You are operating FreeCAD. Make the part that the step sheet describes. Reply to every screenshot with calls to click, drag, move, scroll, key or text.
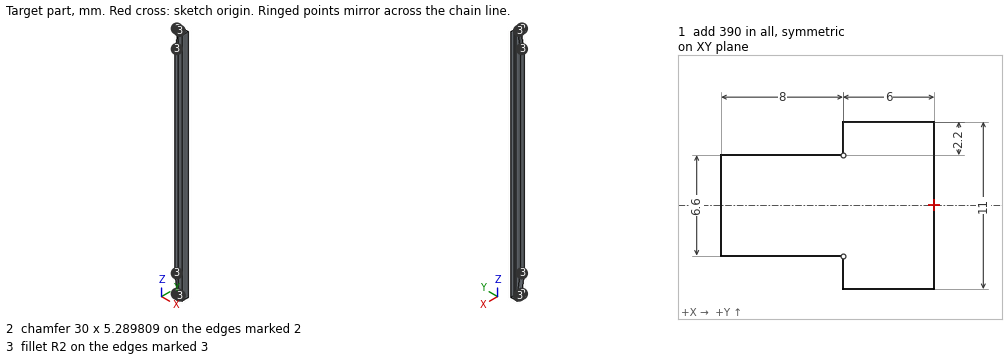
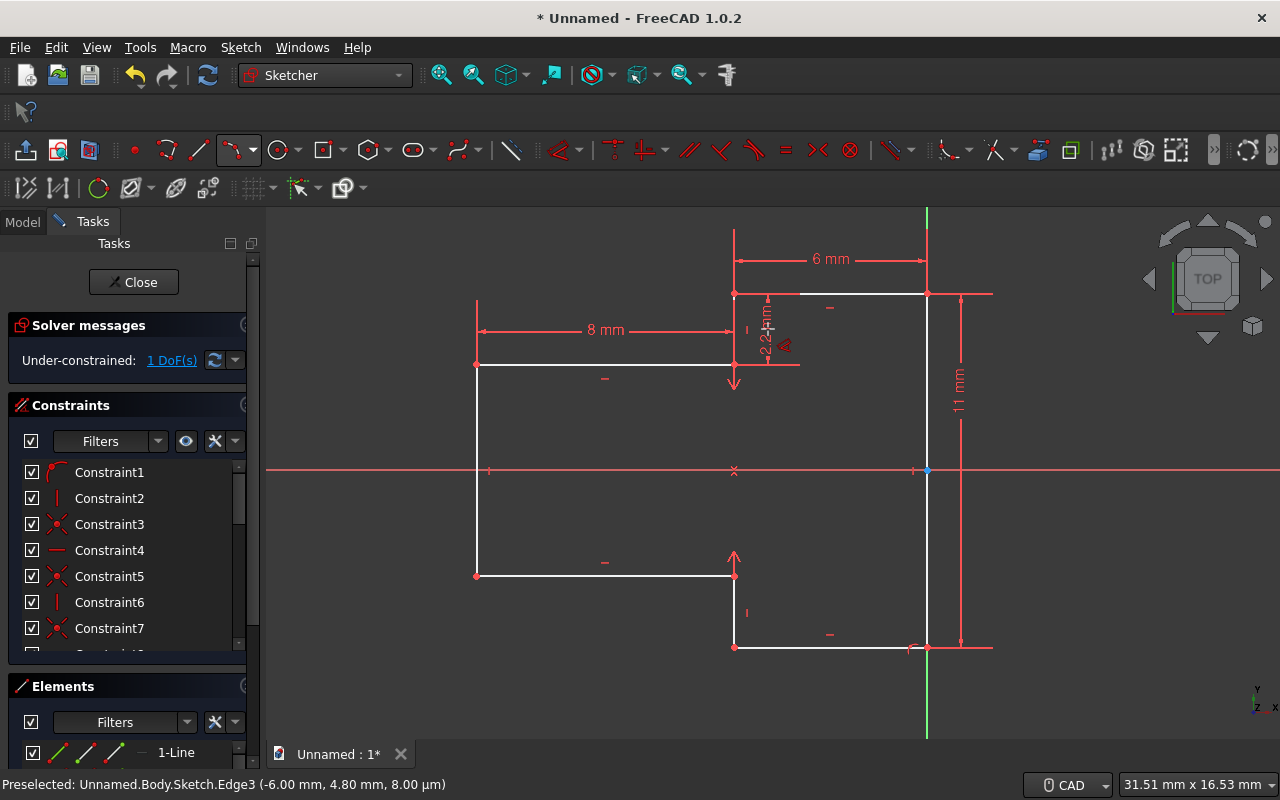
click(477, 428)
click(443, 422)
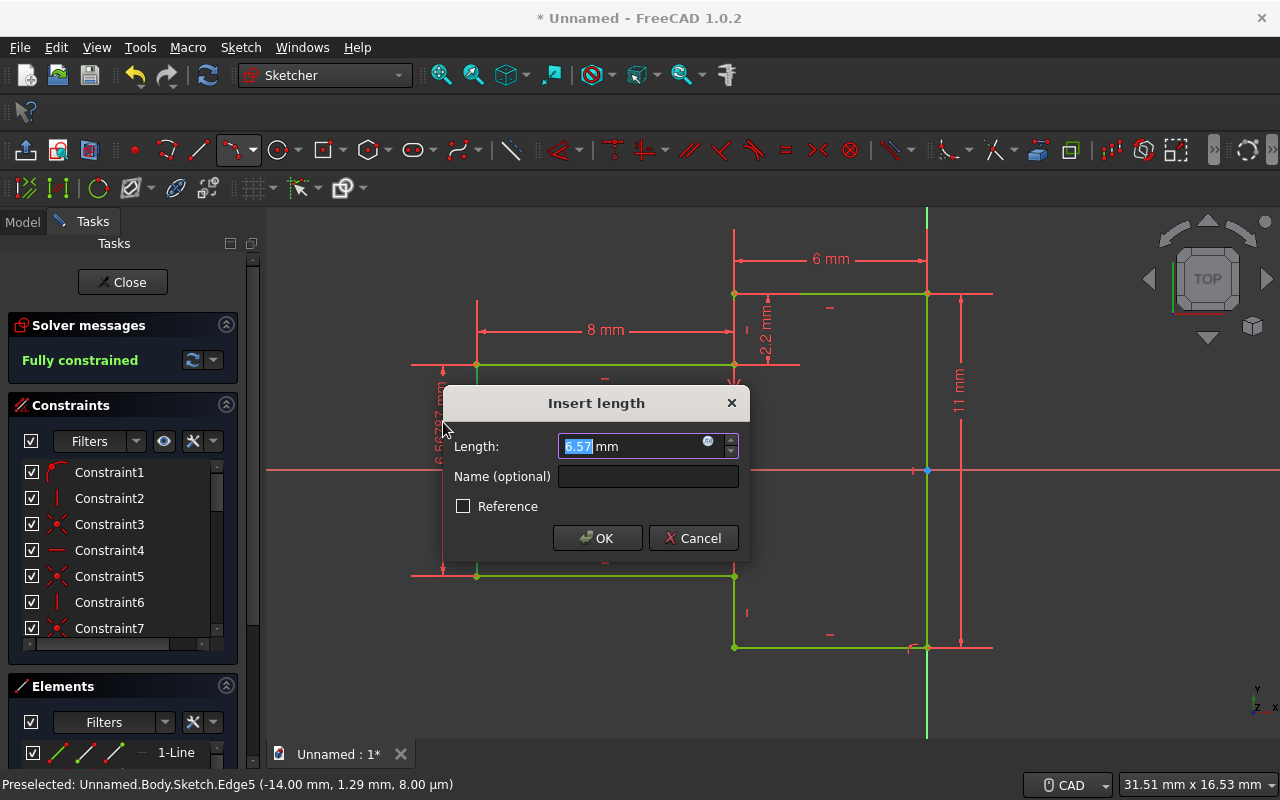
text(6.6)
key(Return)
key(Escape)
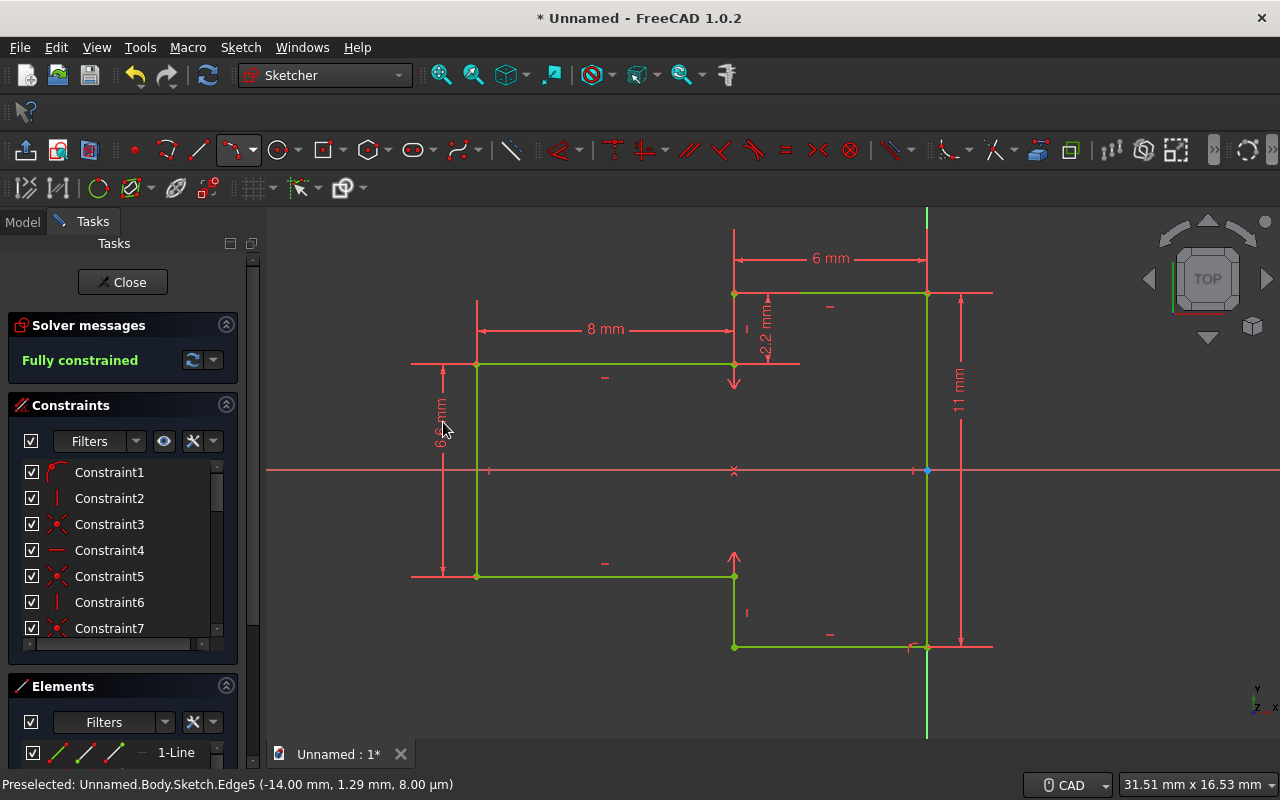
click(123, 282)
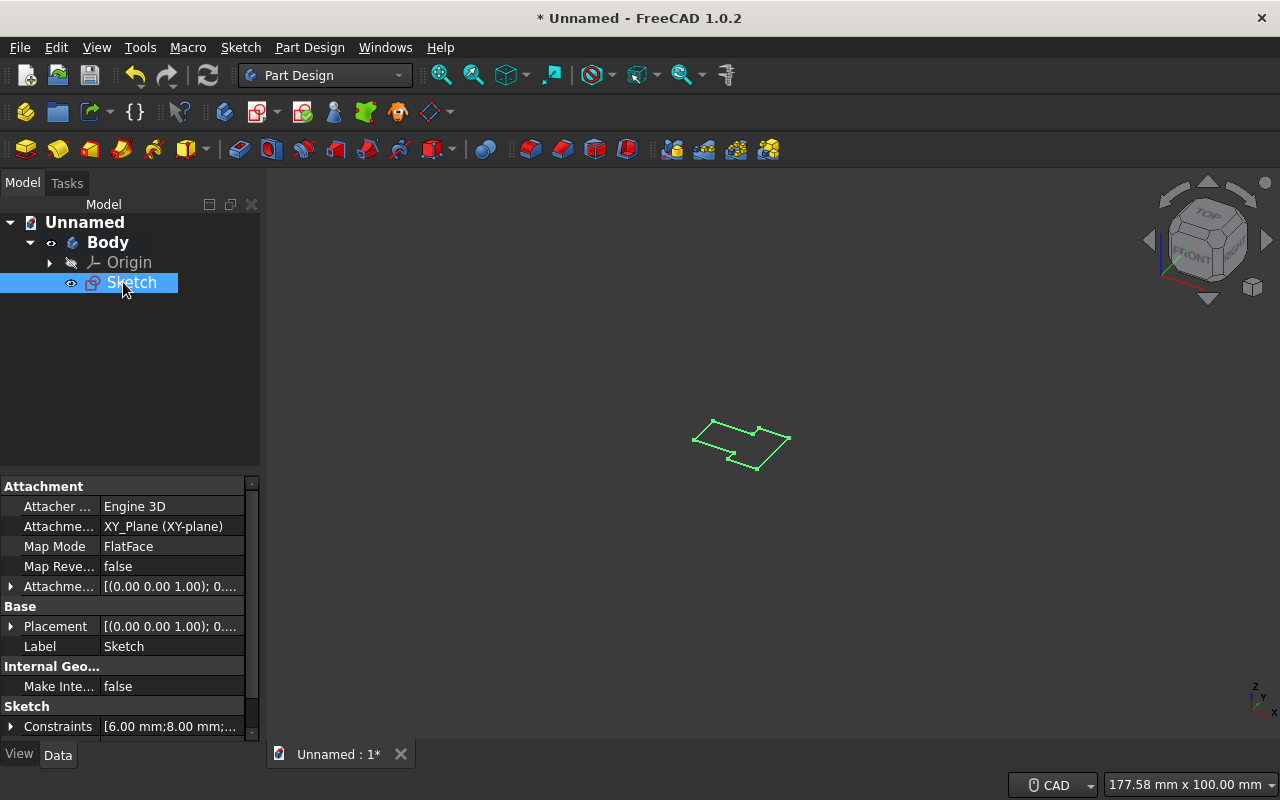
click(26, 150)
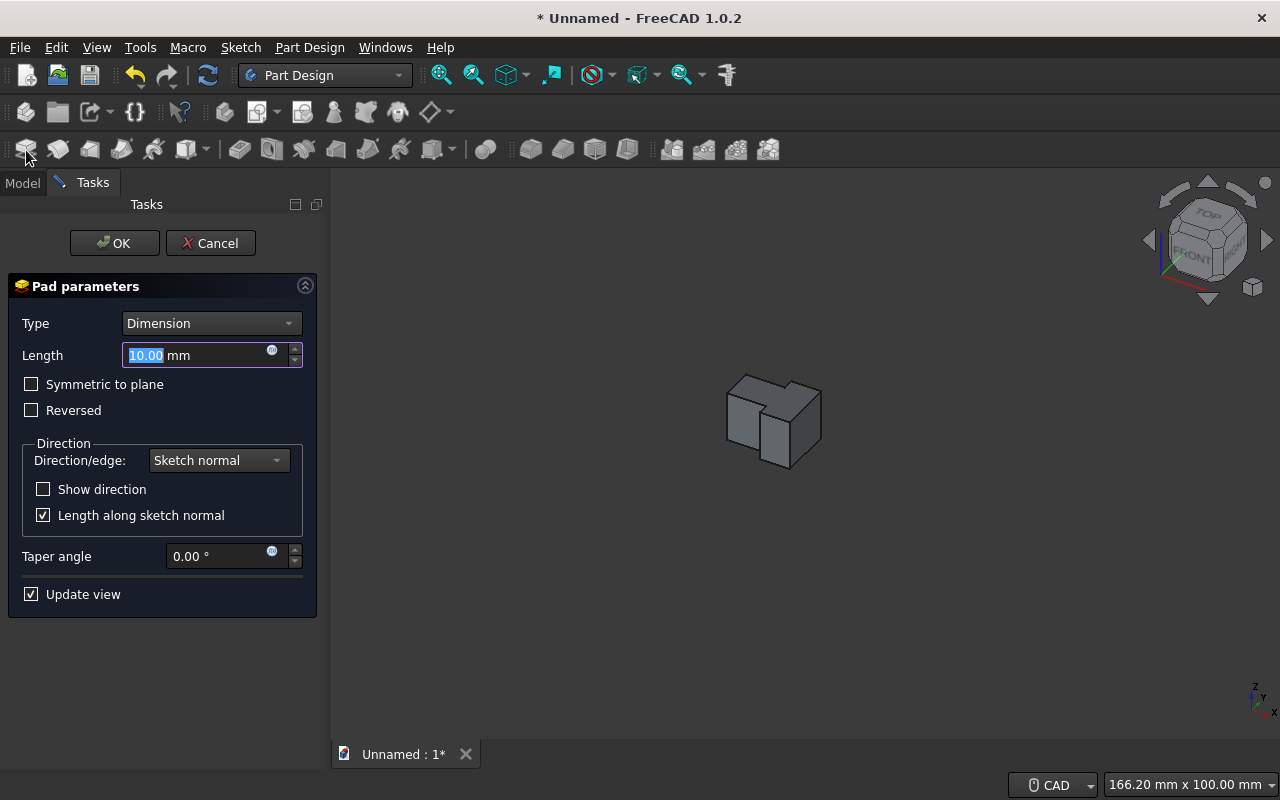
text(390)
key(Tab)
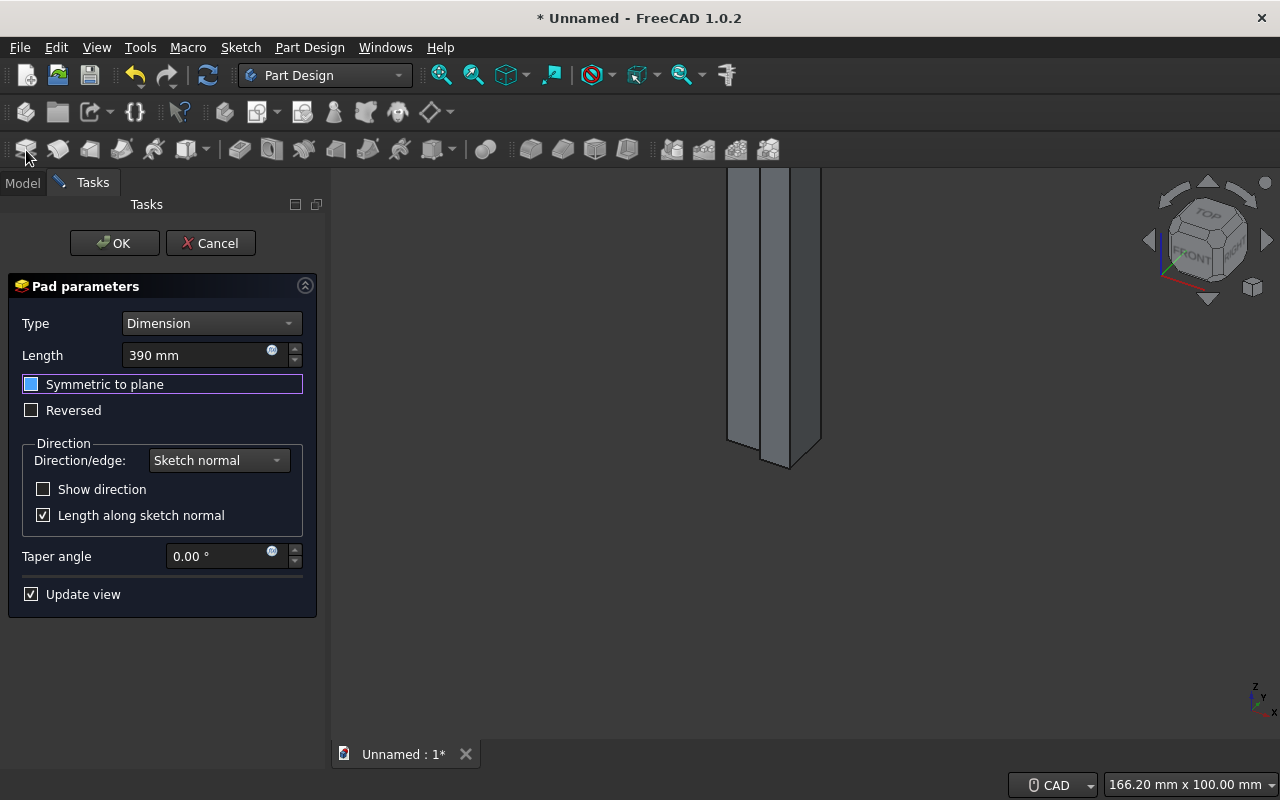
click(30, 384)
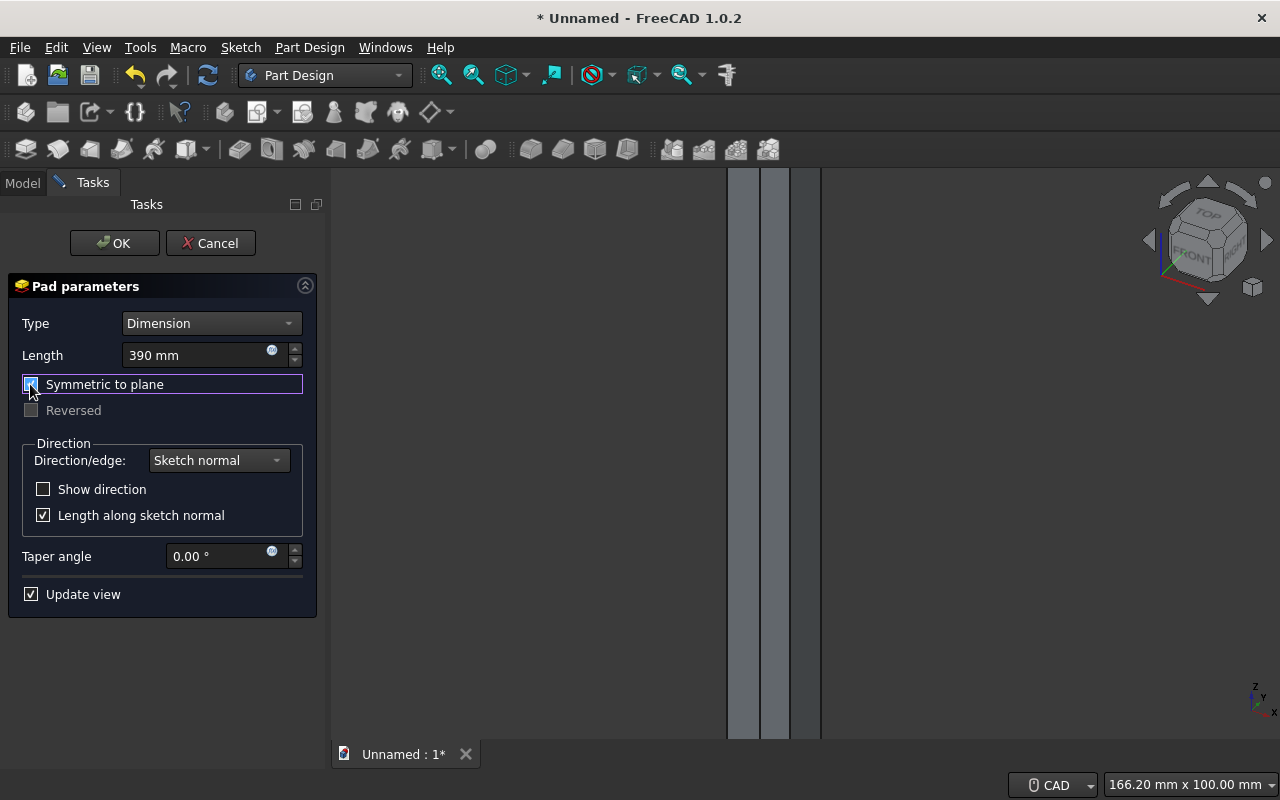
click(115, 243)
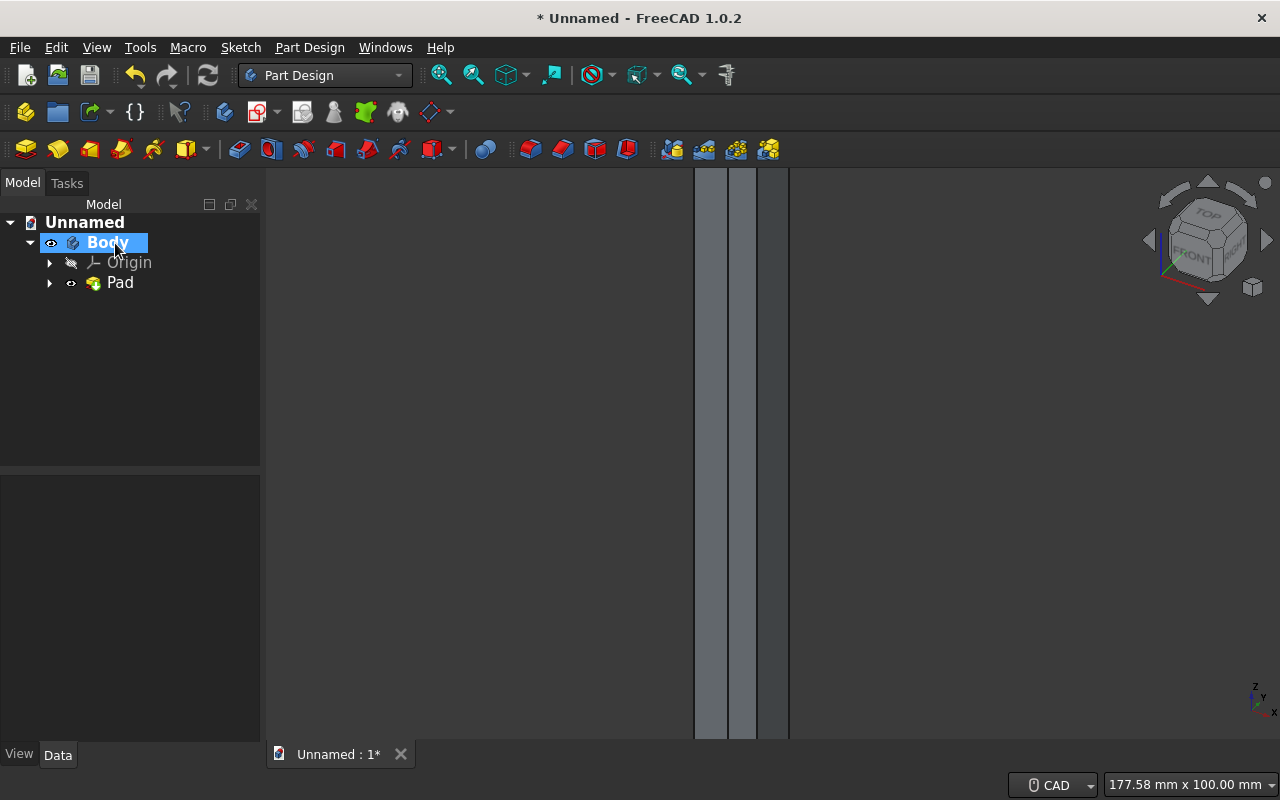
click(442, 76)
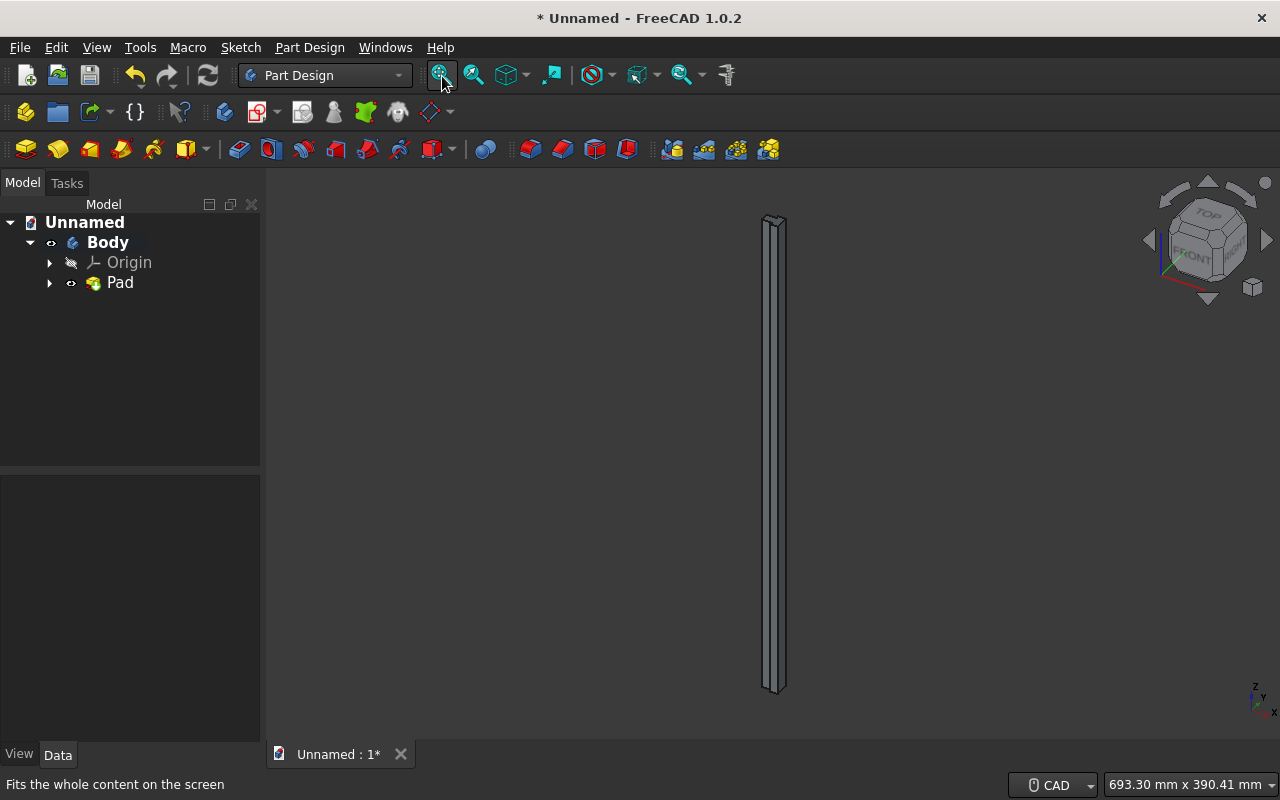
scroll(764, 216, up, 8)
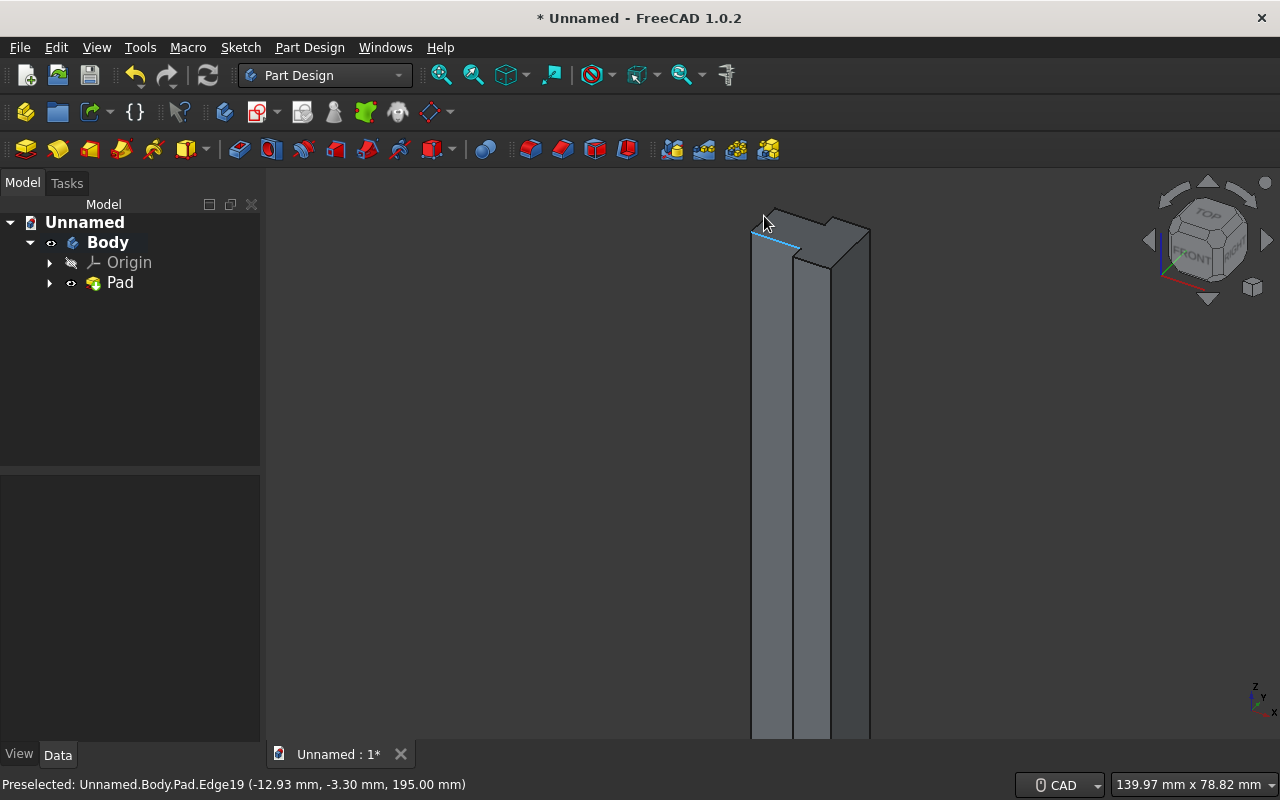
click(442, 76)